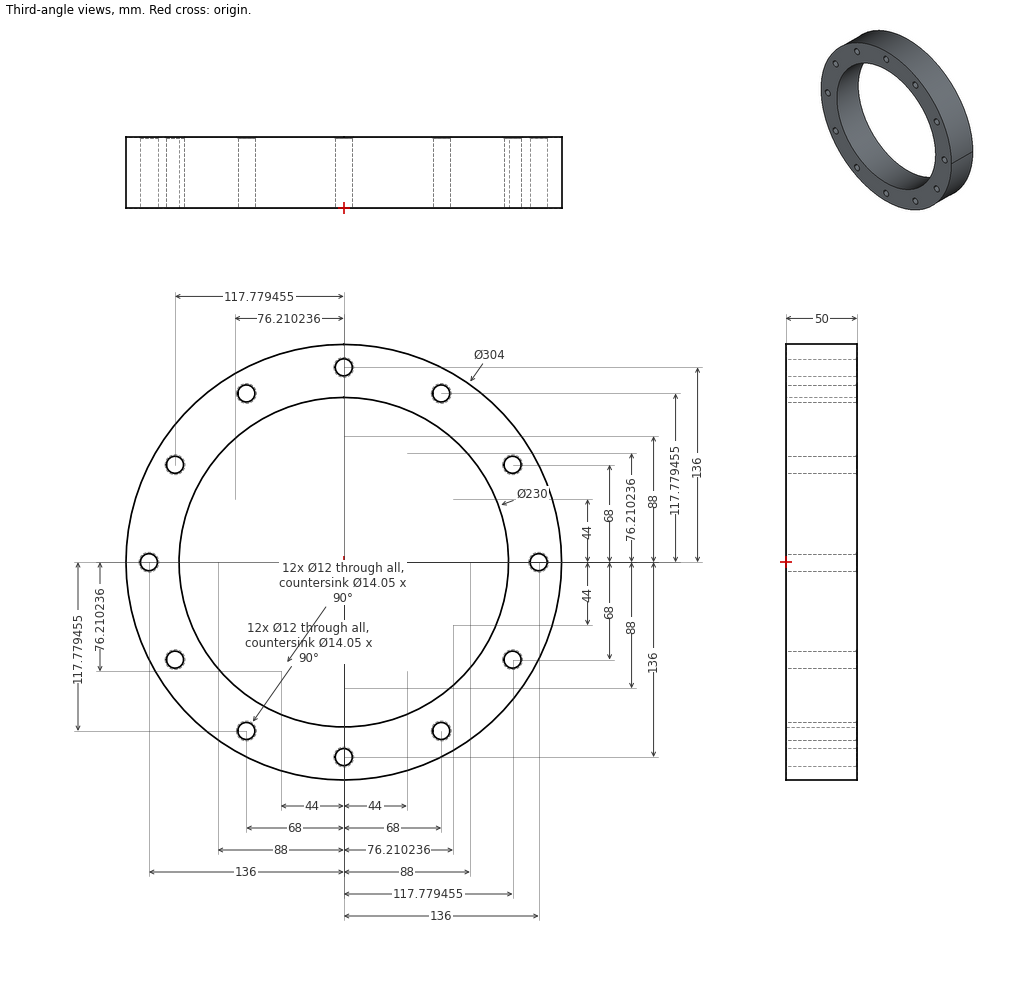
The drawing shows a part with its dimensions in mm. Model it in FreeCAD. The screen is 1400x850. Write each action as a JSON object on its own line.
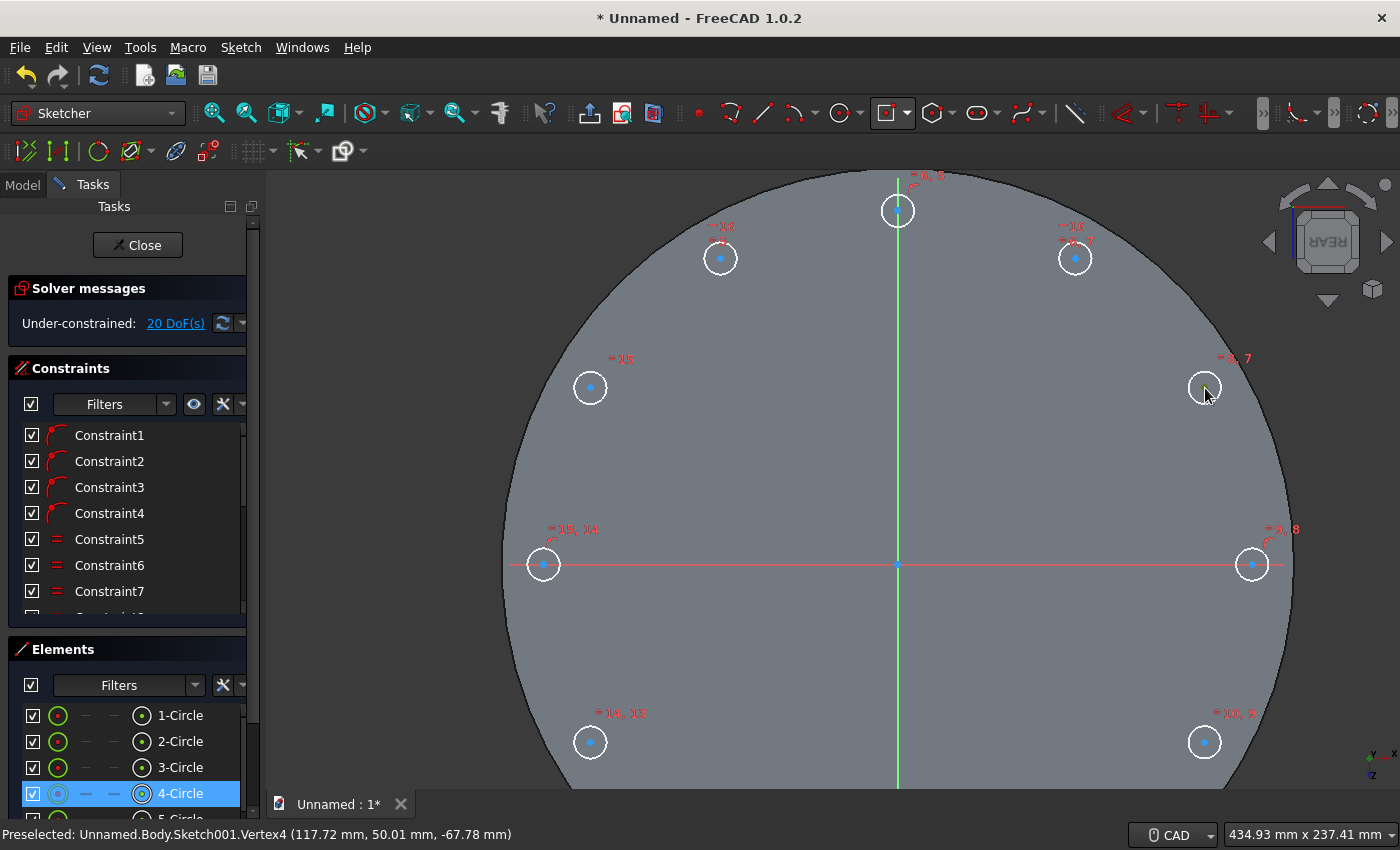
{"action": "left_click", "coordinate": [1205, 742]}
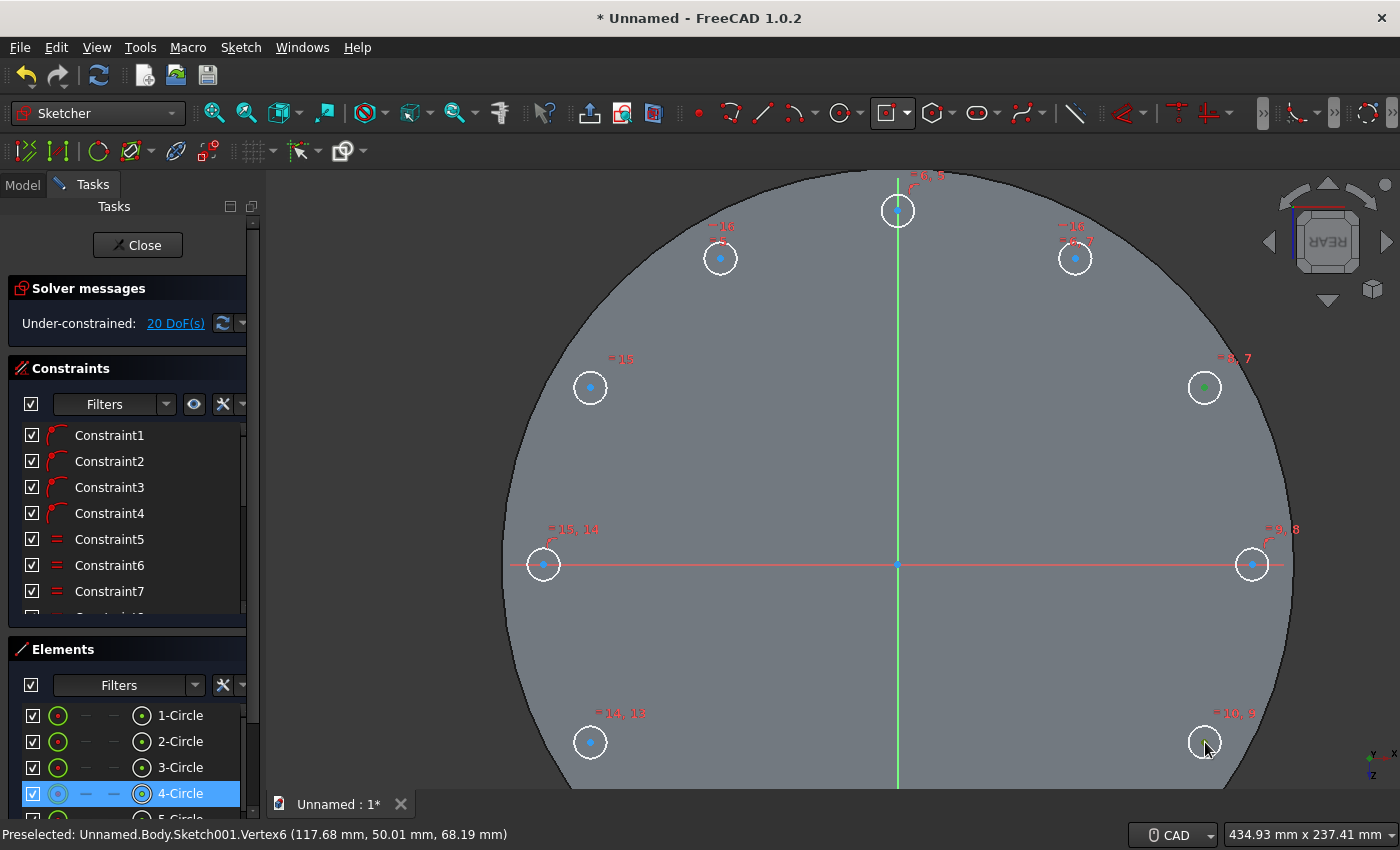
{"action": "left_click", "coordinate": [1232, 114]}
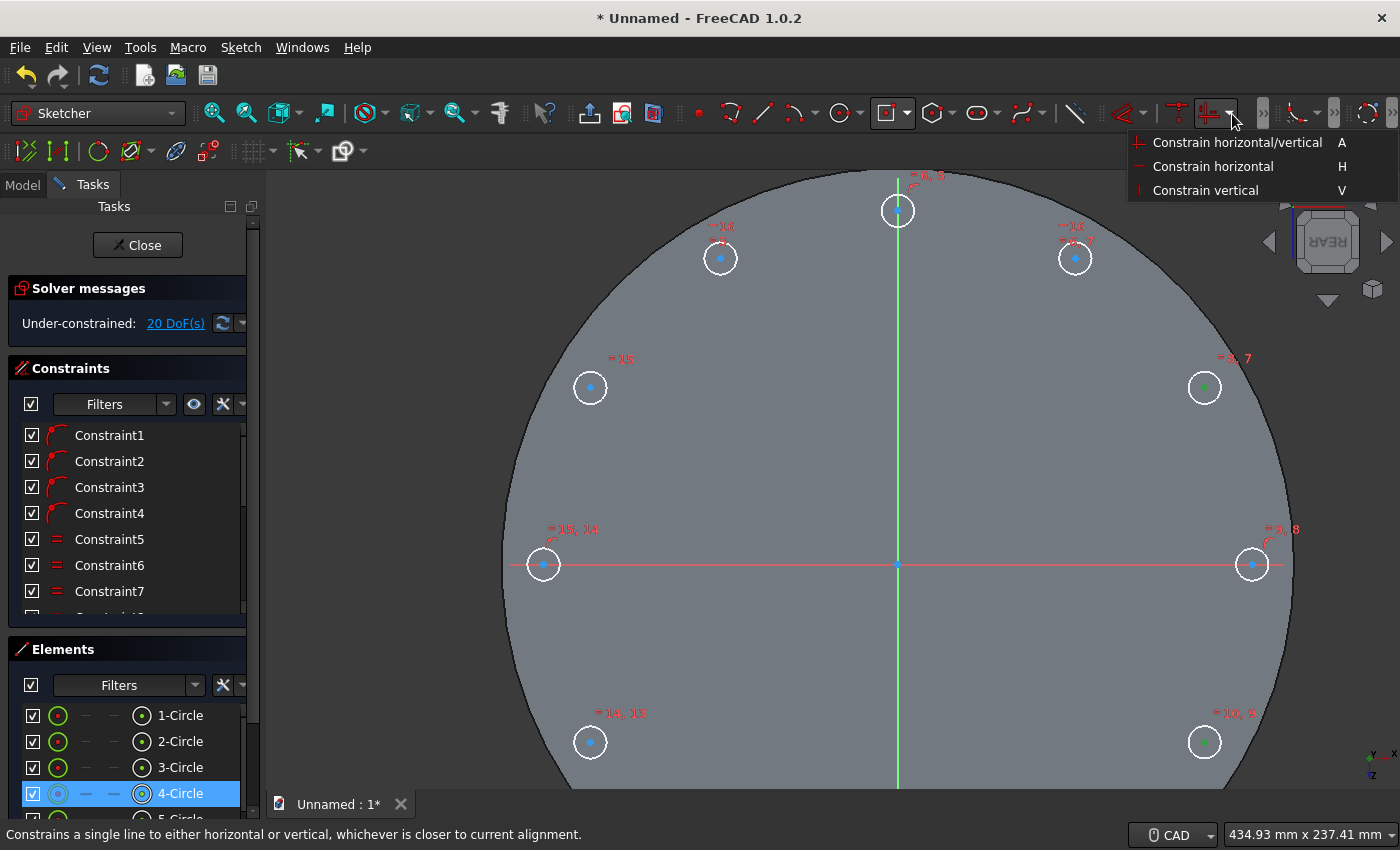
{"action": "left_click", "coordinate": [1263, 190]}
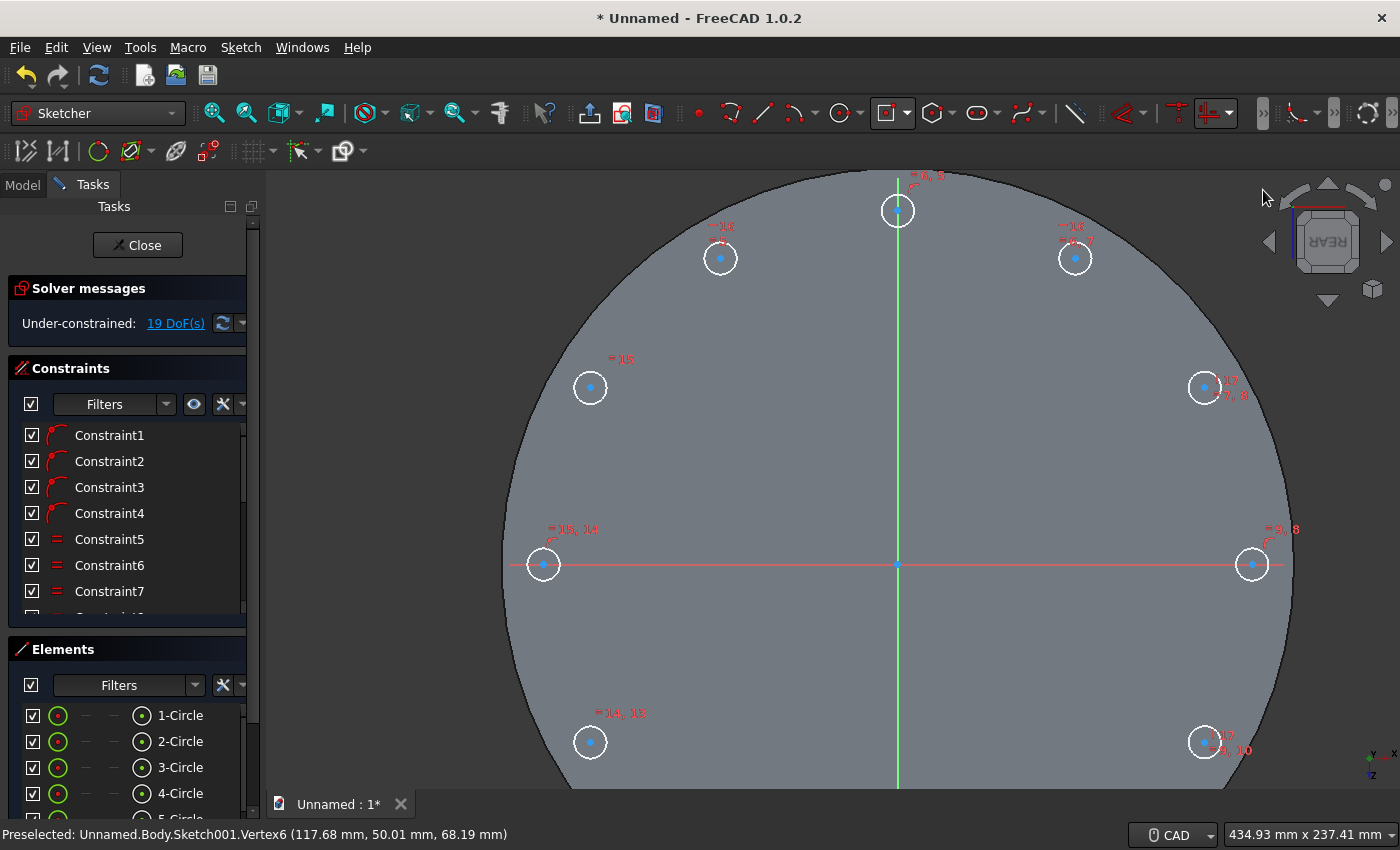
{"action": "left_click", "coordinate": [1075, 258]}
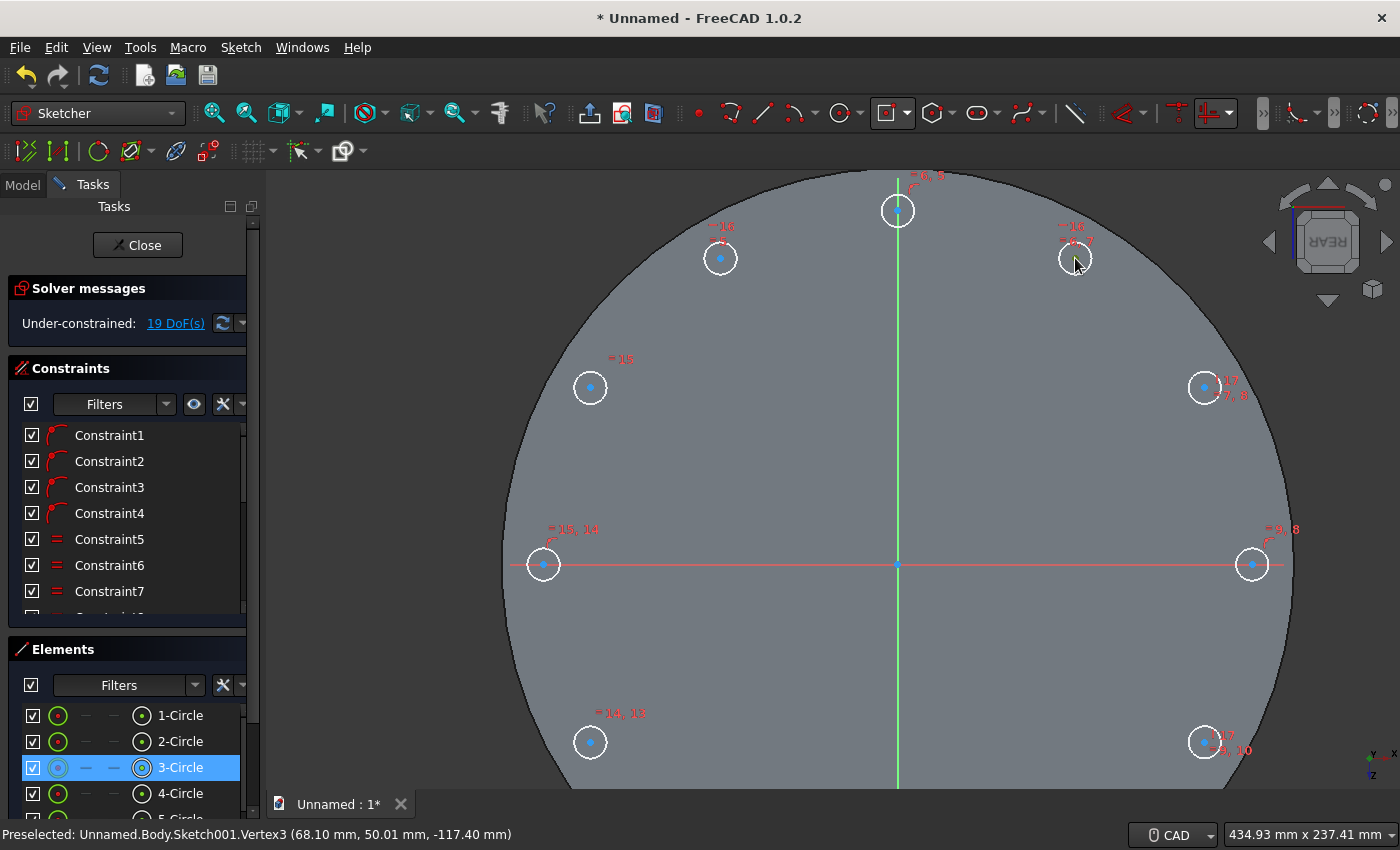
{"action": "scroll", "coordinate": [602, 376], "scroll_direction": "down", "scroll_amount": 3}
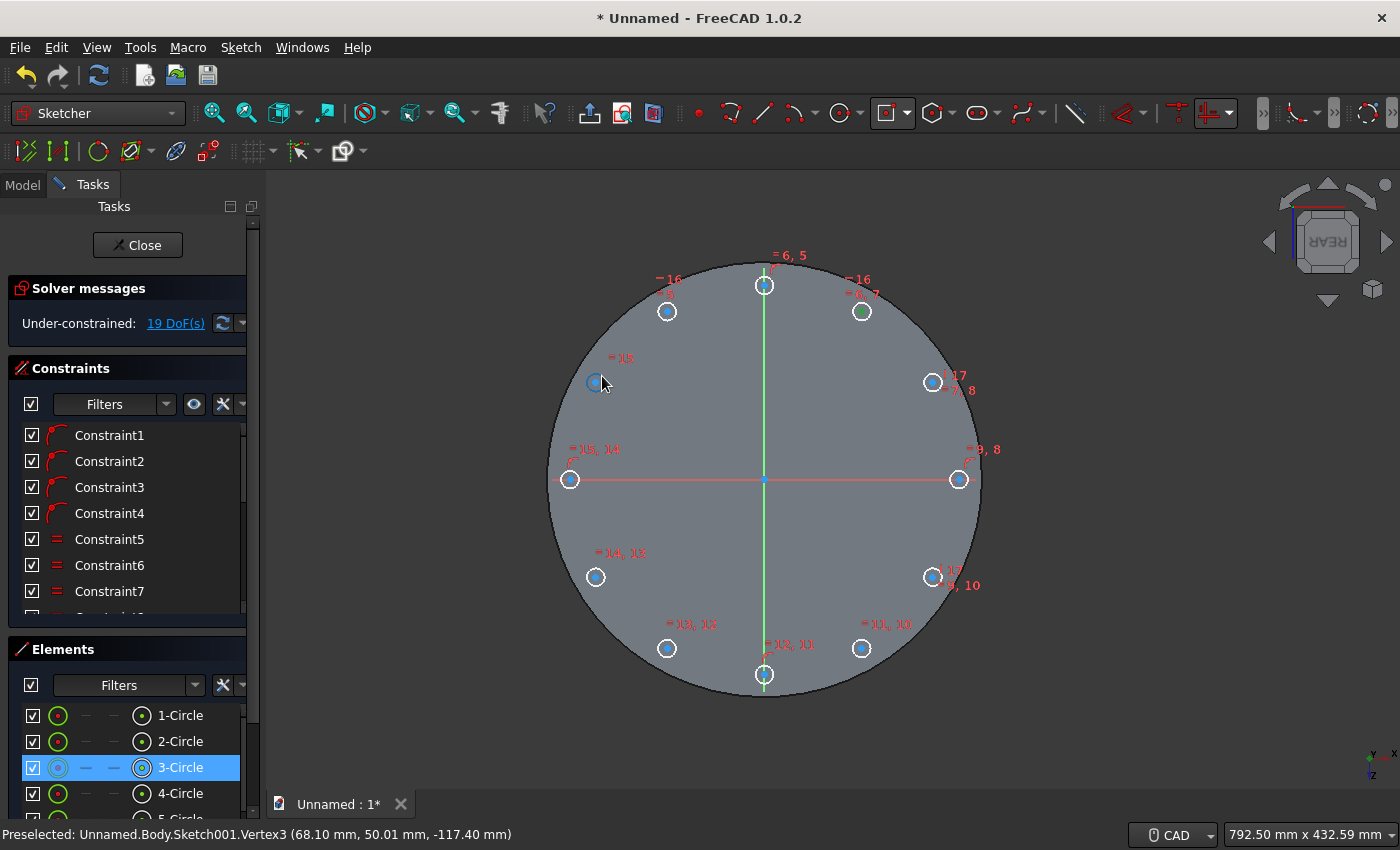
{"action": "left_click", "coordinate": [862, 649]}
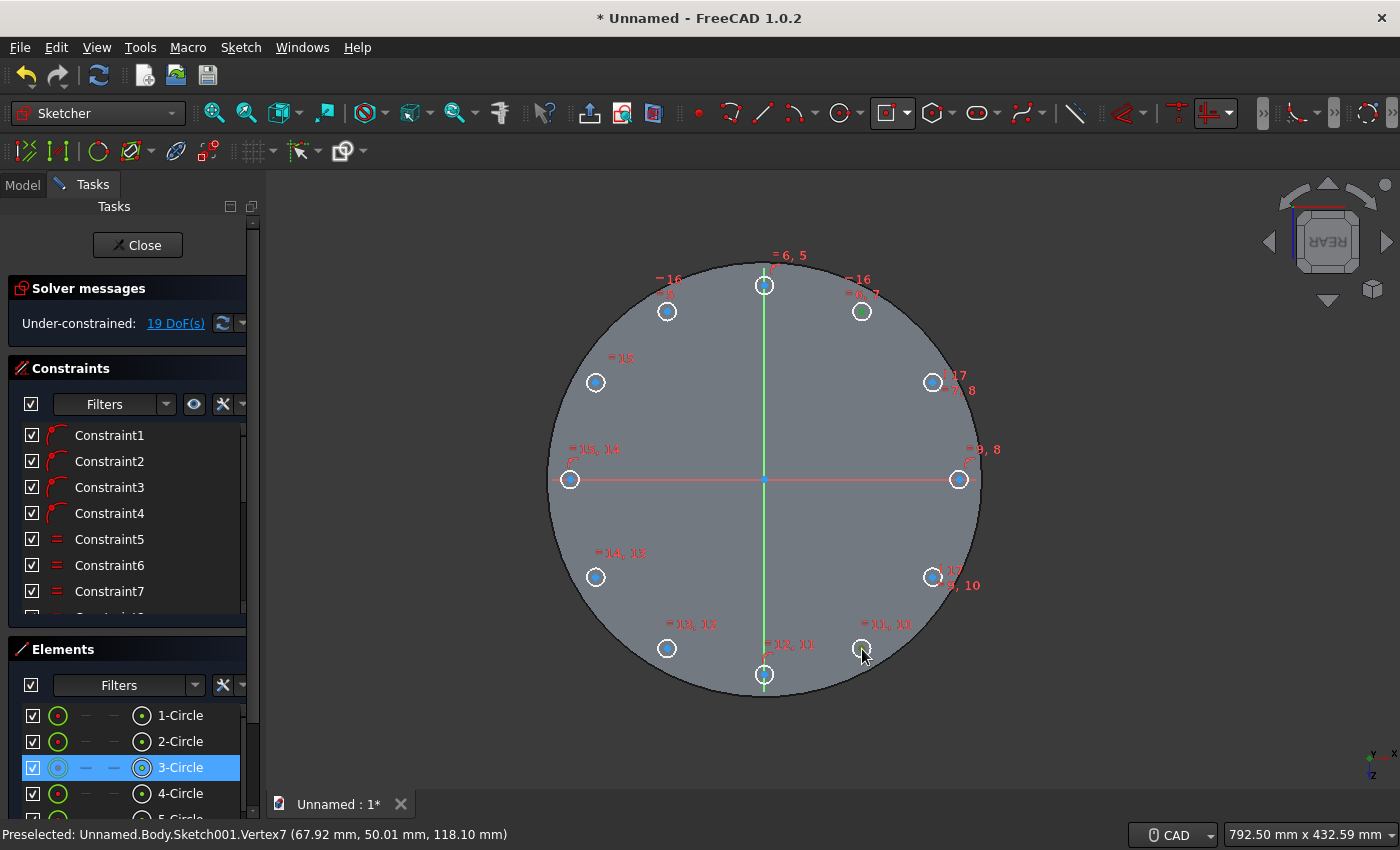
{"action": "left_click", "coordinate": [1232, 114]}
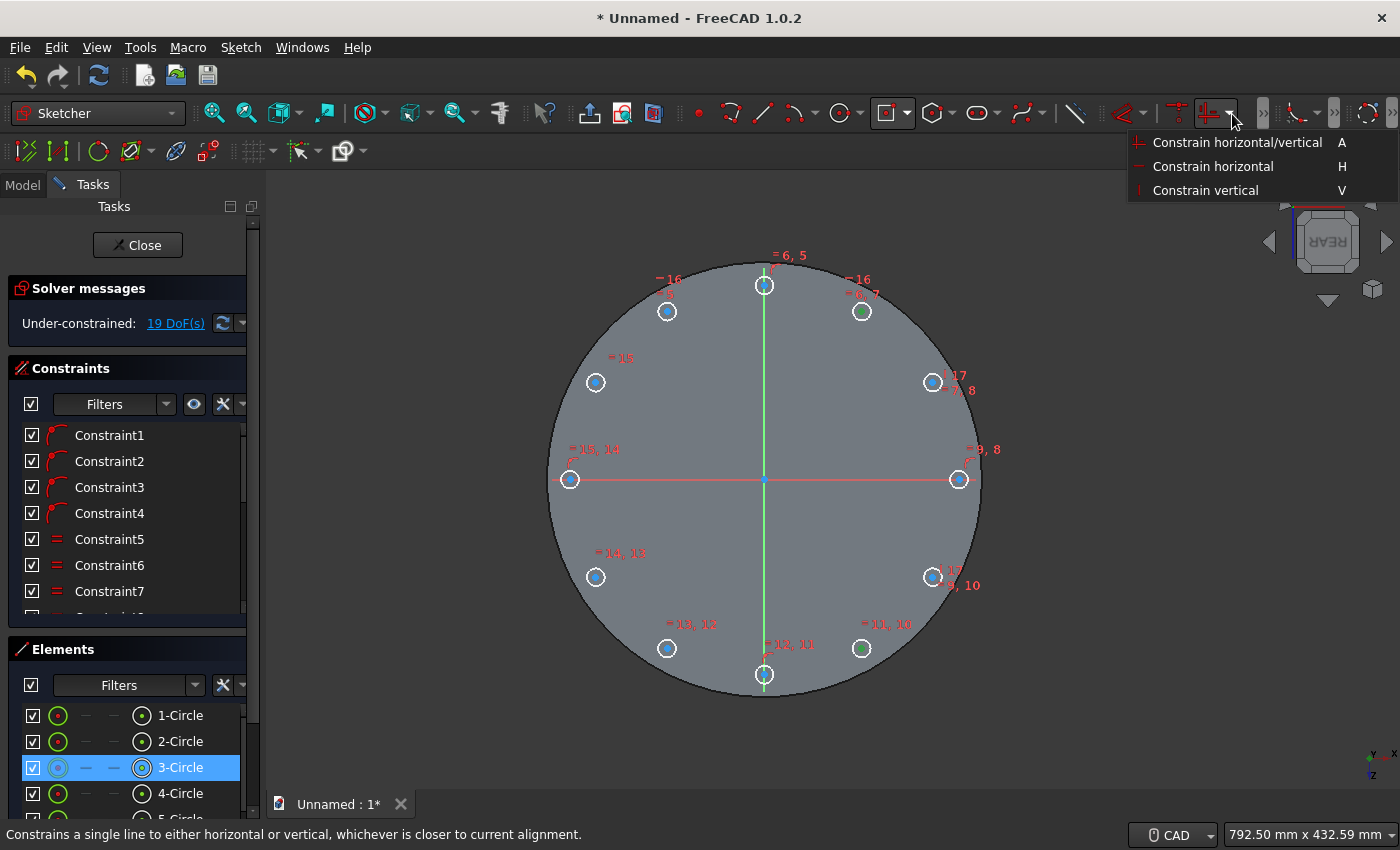
{"action": "left_click", "coordinate": [1263, 190]}